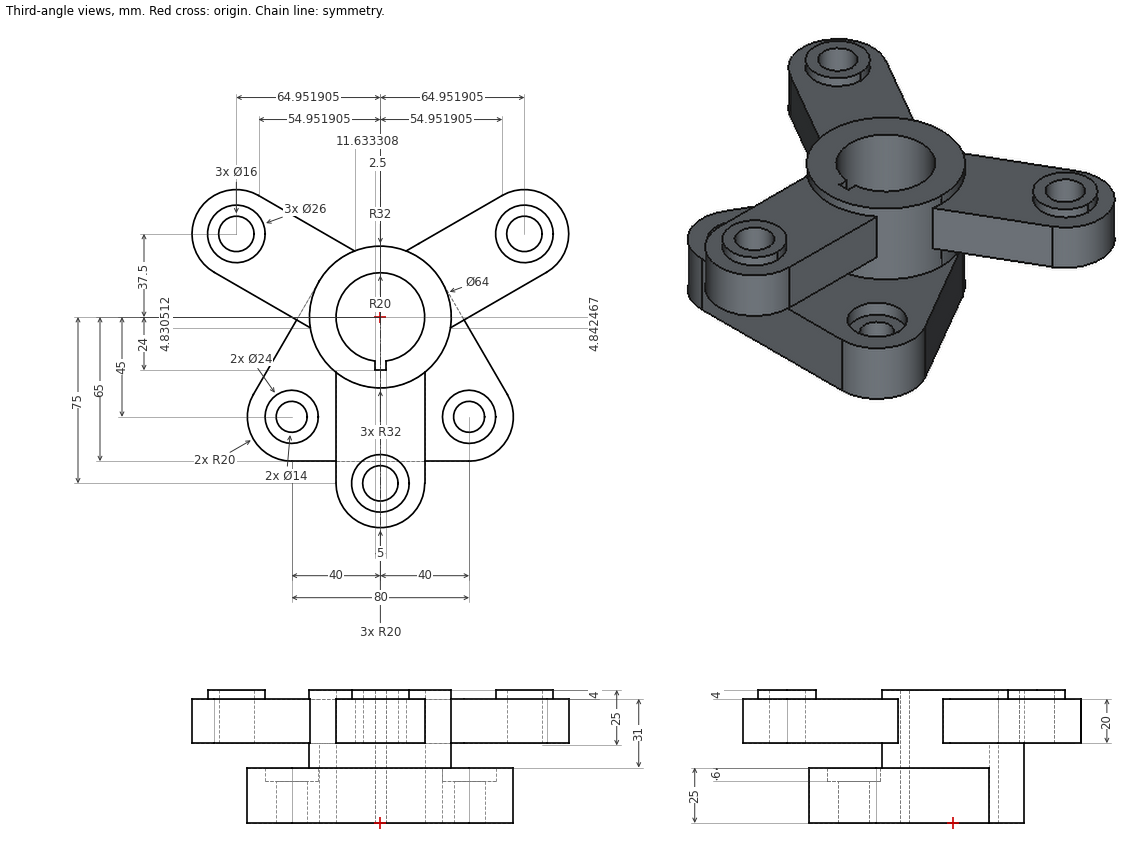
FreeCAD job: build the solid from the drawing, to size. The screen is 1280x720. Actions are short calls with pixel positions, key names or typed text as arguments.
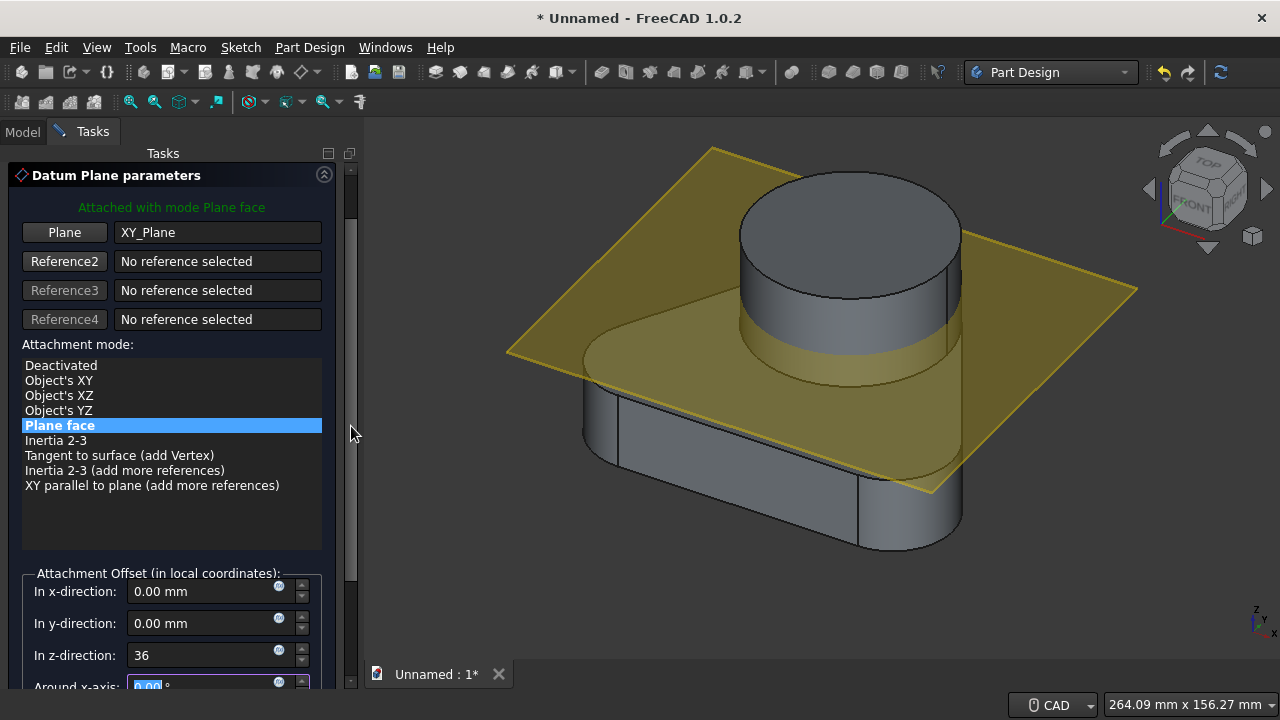
click(124, 192)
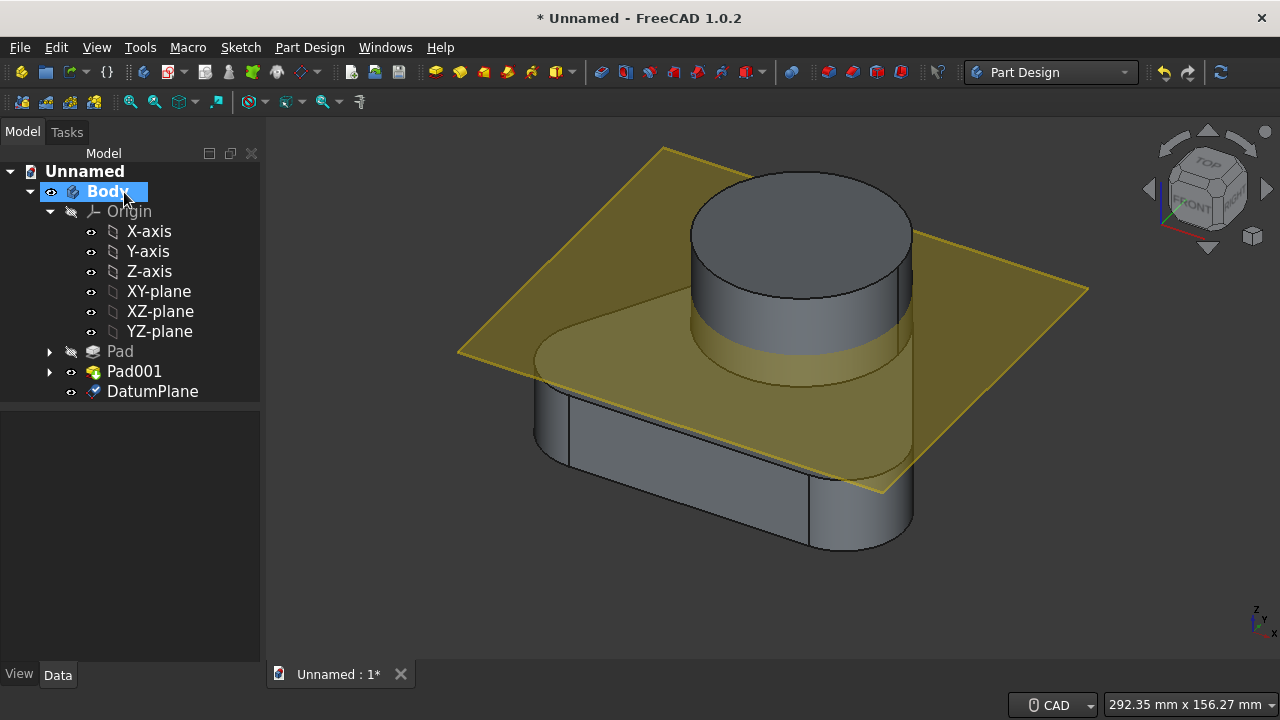
click(116, 392)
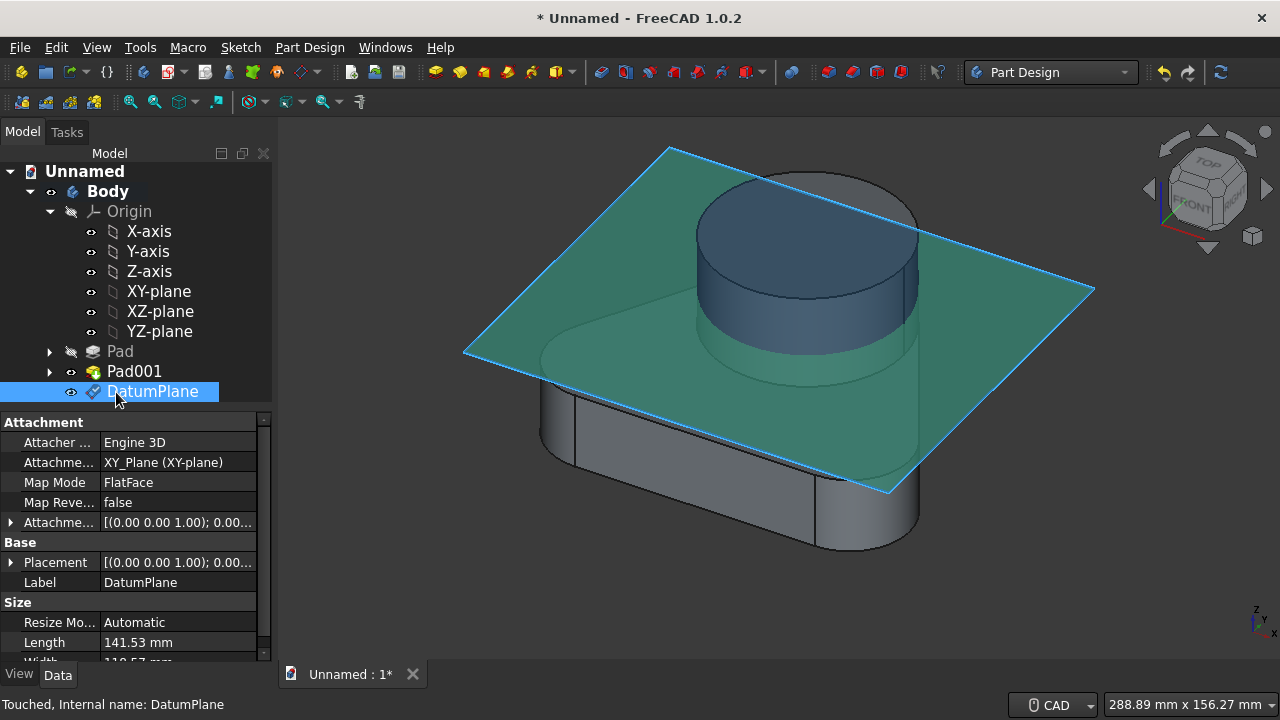
click(168, 72)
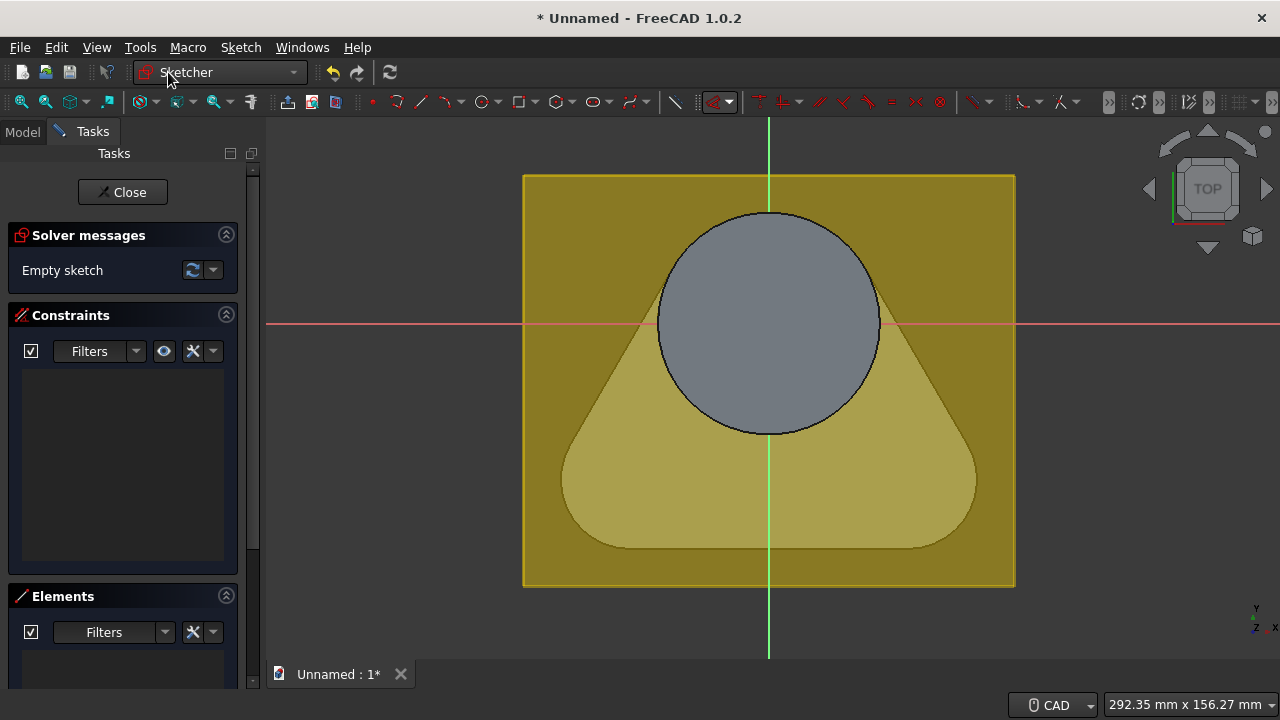
click(336, 102)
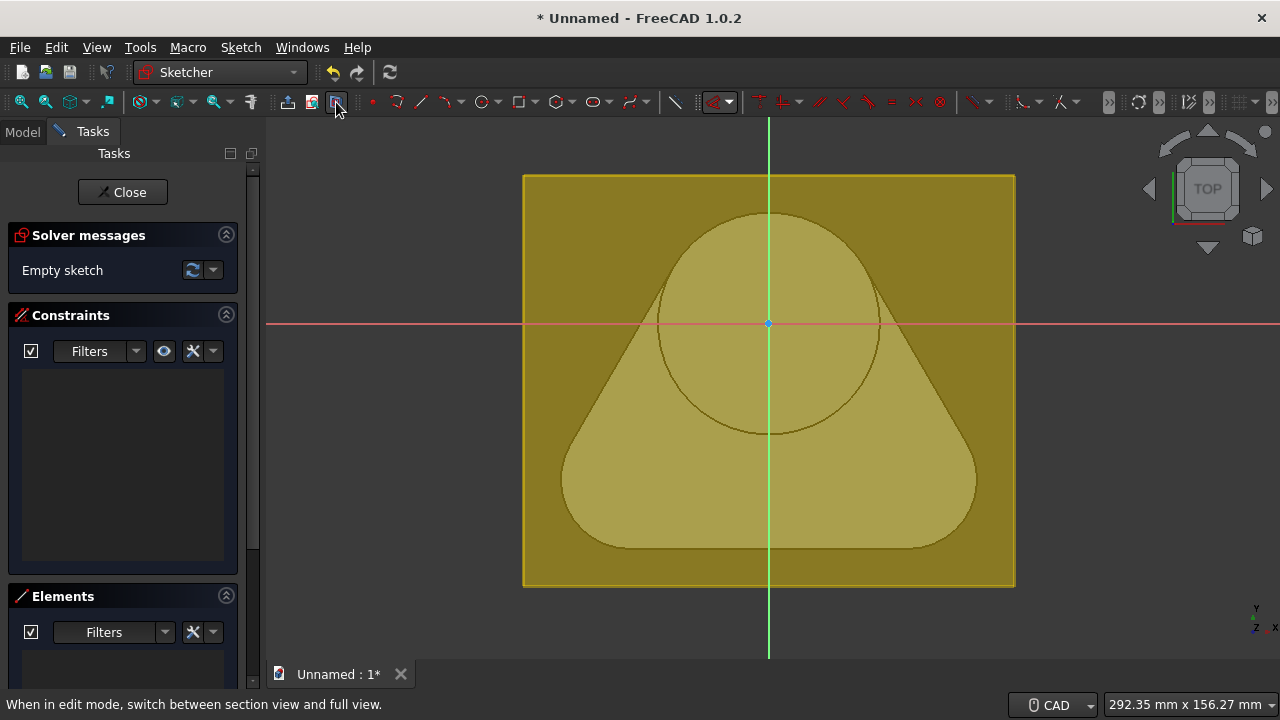
scroll(573, 377, down, 2)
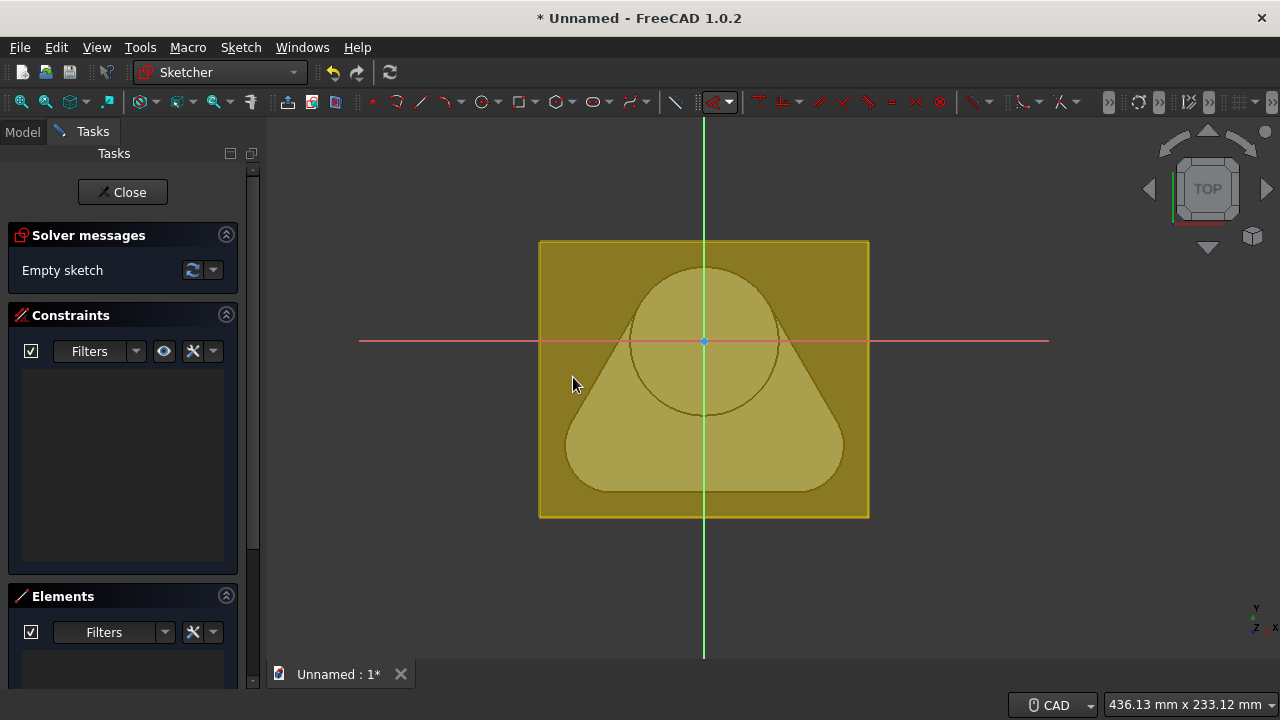
click(422, 102)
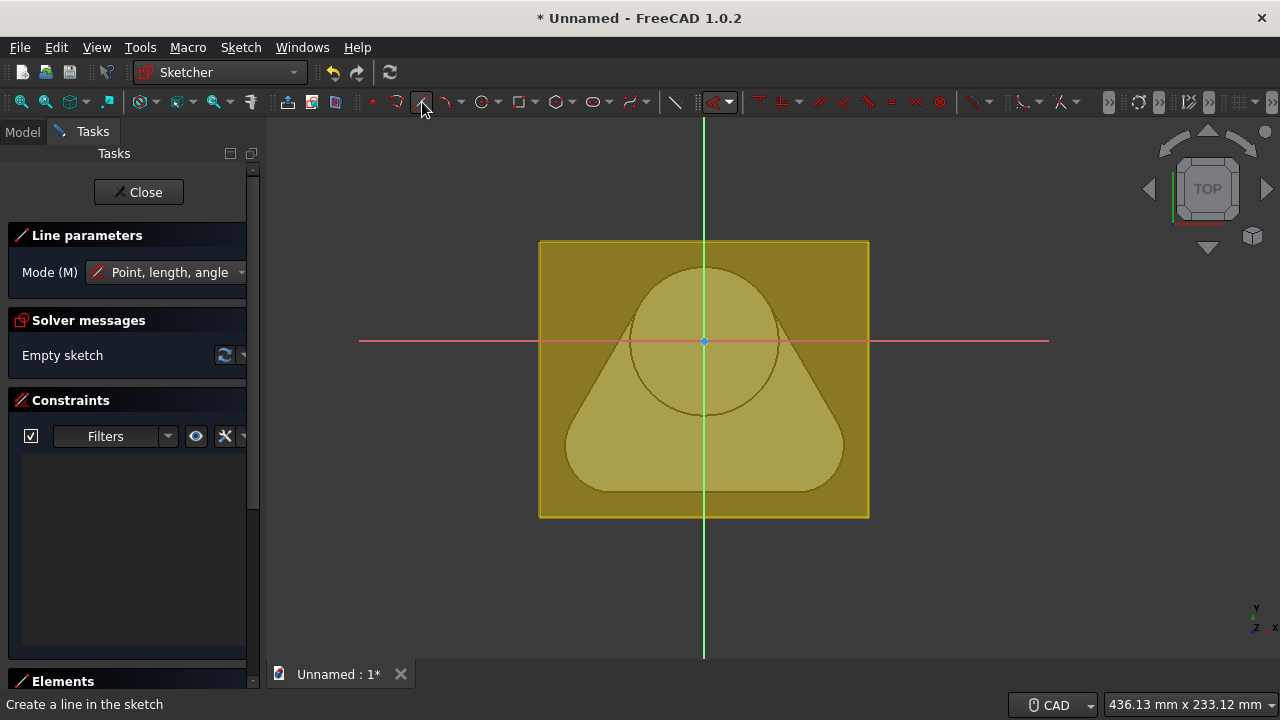
click(658, 399)
click(658, 516)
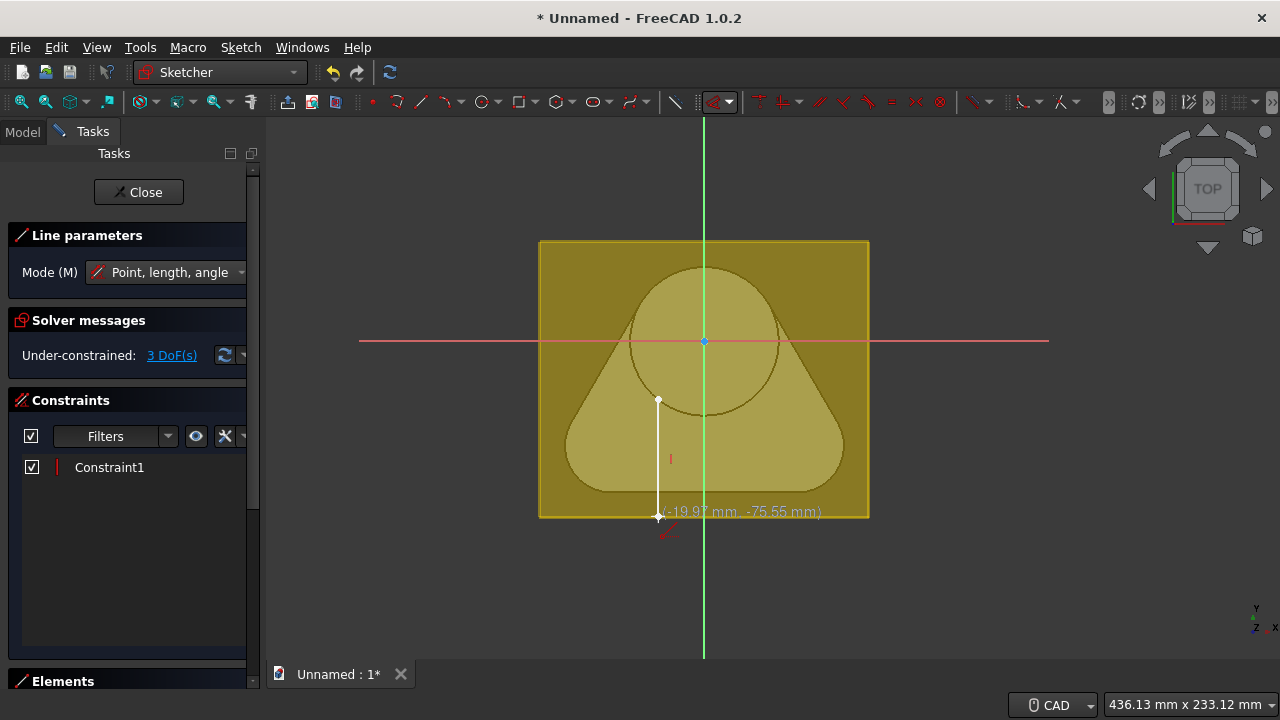
click(751, 516)
click(751, 399)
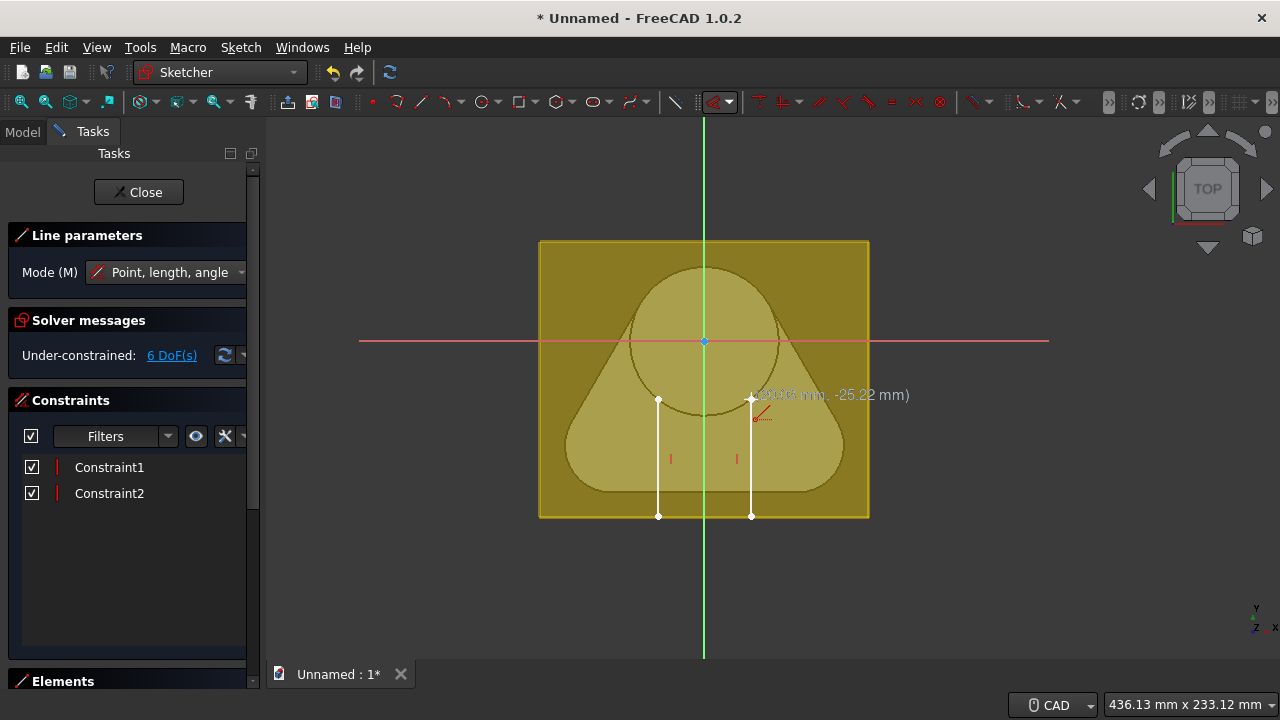
click(446, 102)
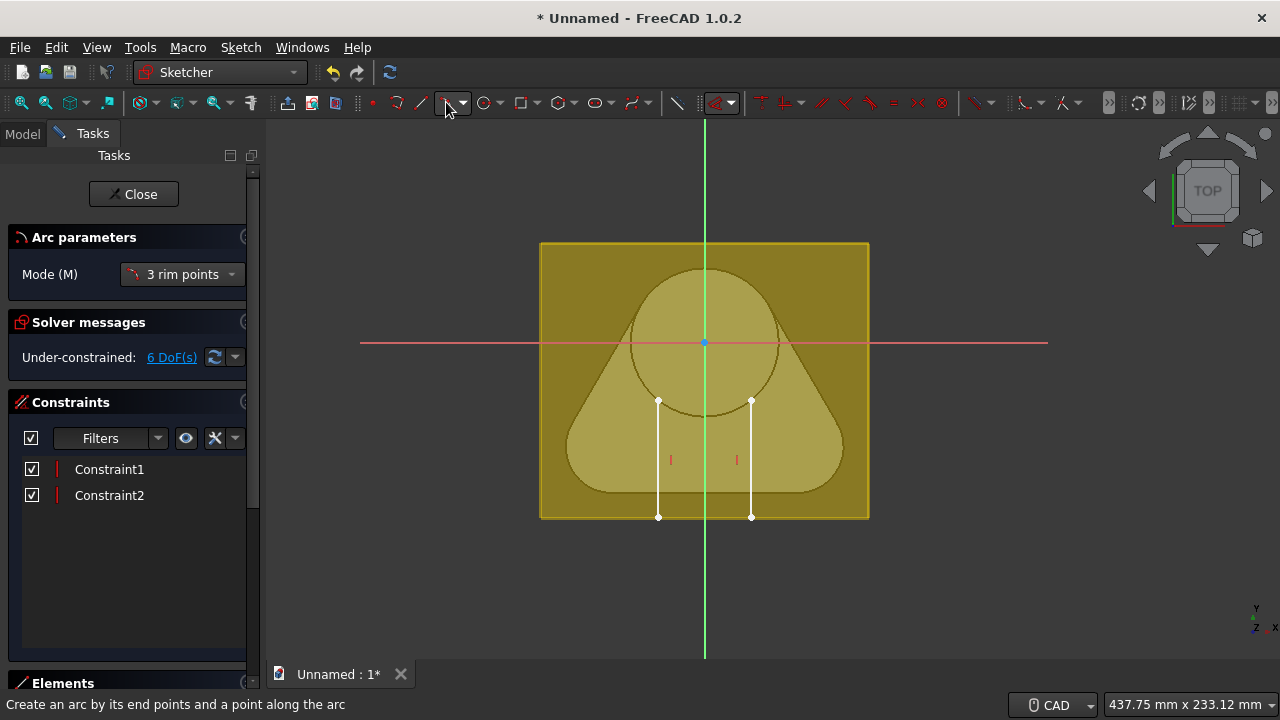
click(658, 518)
click(751, 518)
click(690, 560)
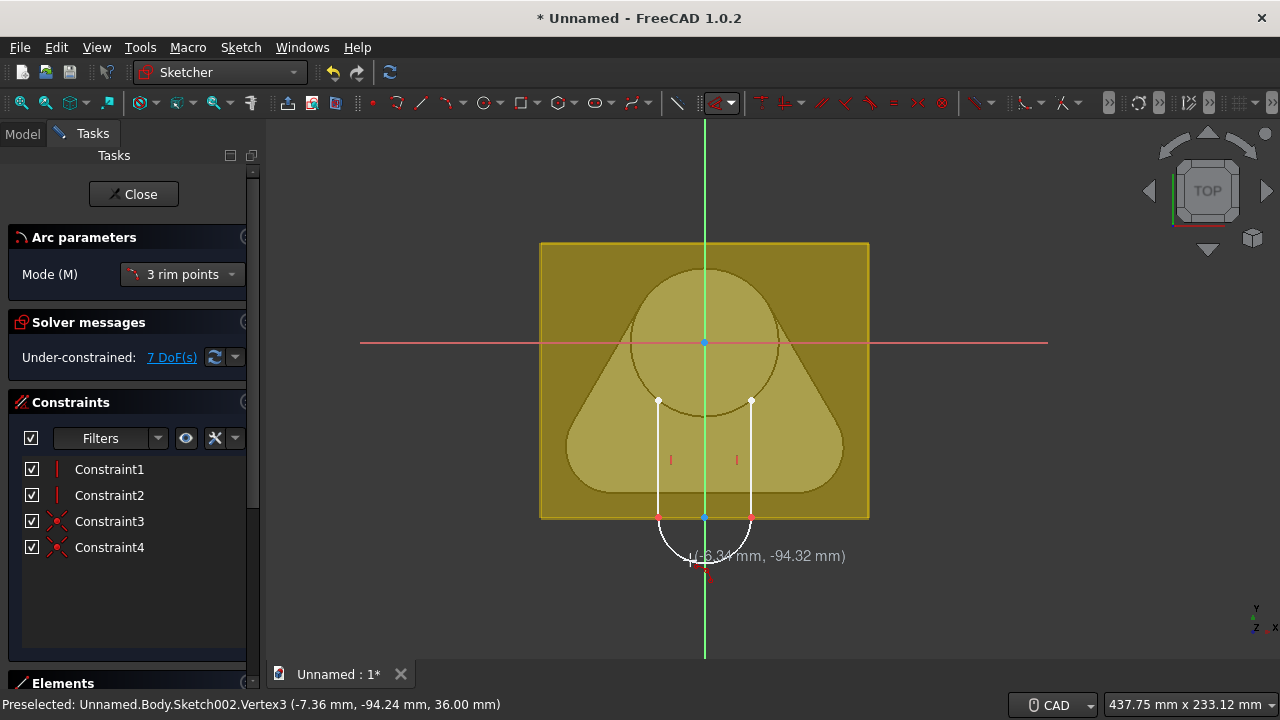
click(751, 401)
click(658, 401)
click(685, 414)